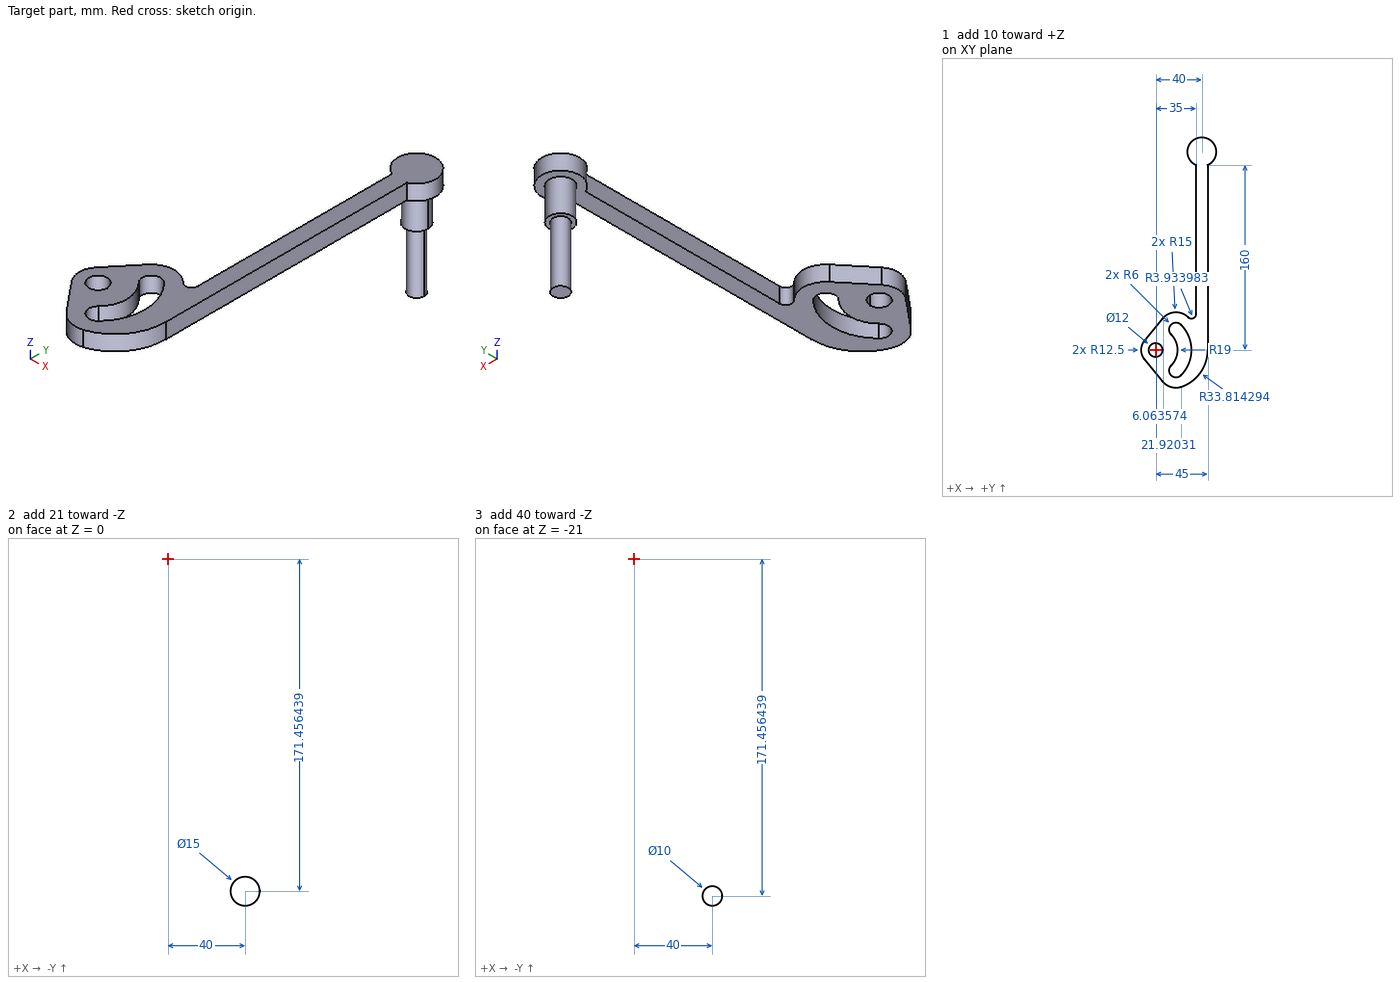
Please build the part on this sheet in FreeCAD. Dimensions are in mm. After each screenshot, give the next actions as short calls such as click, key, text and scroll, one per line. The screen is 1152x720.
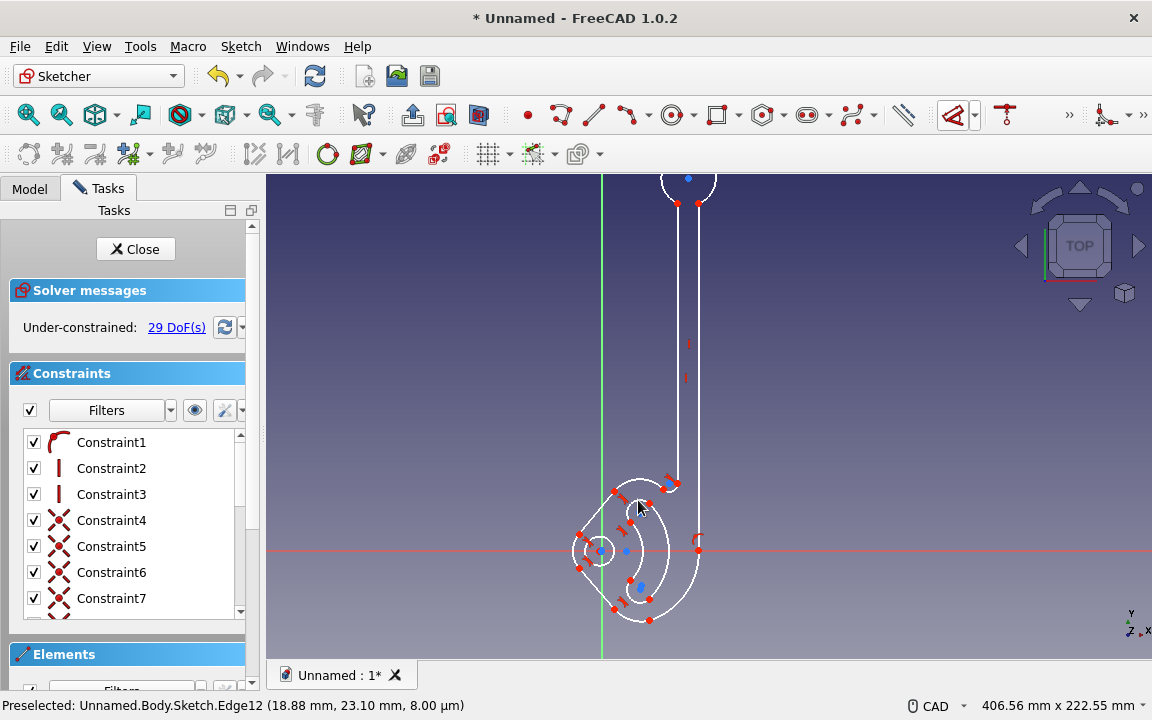
click(641, 564)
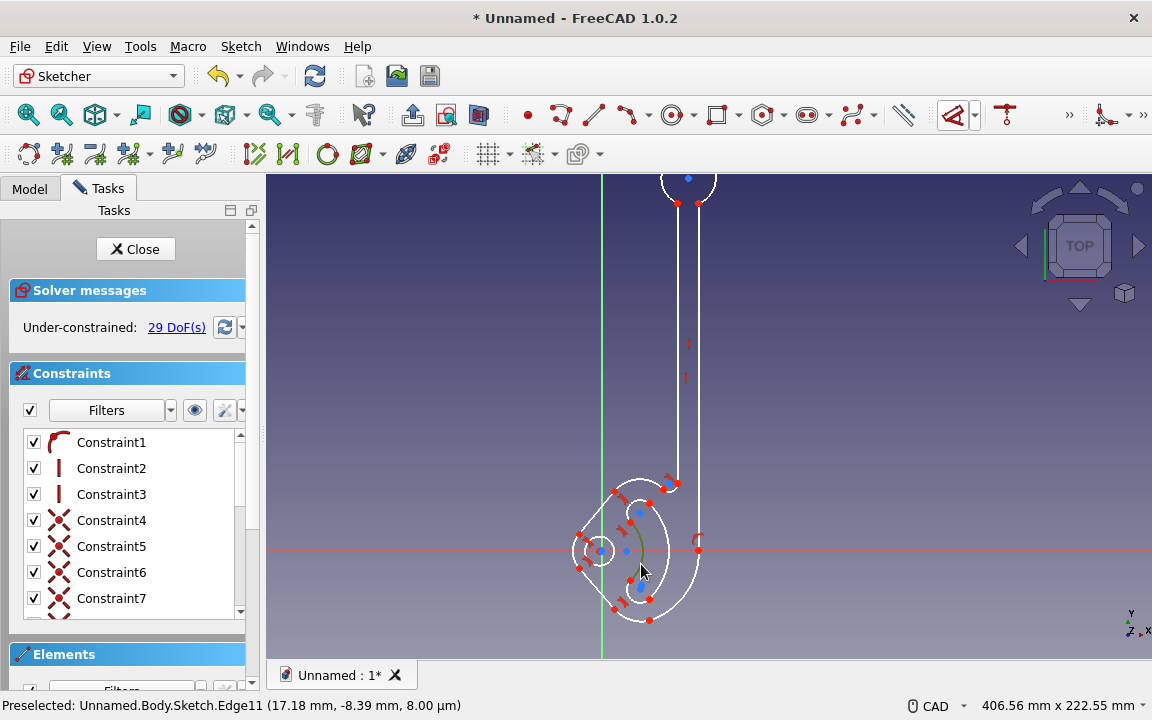
click(627, 592)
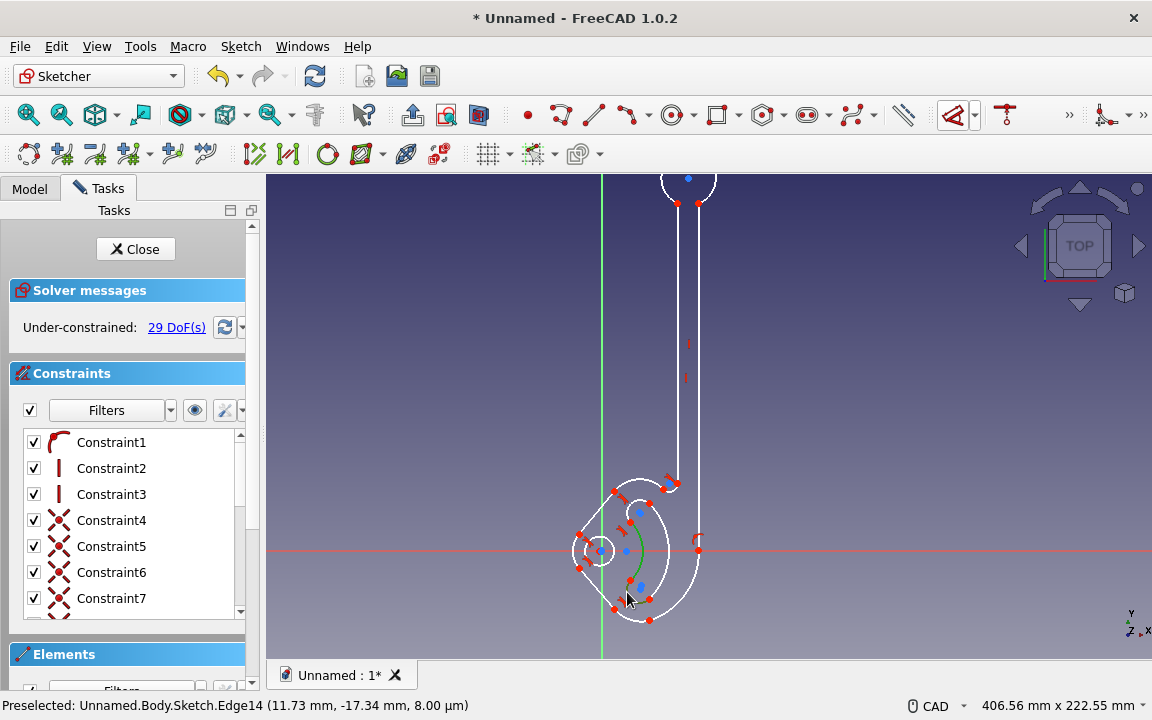
key(t)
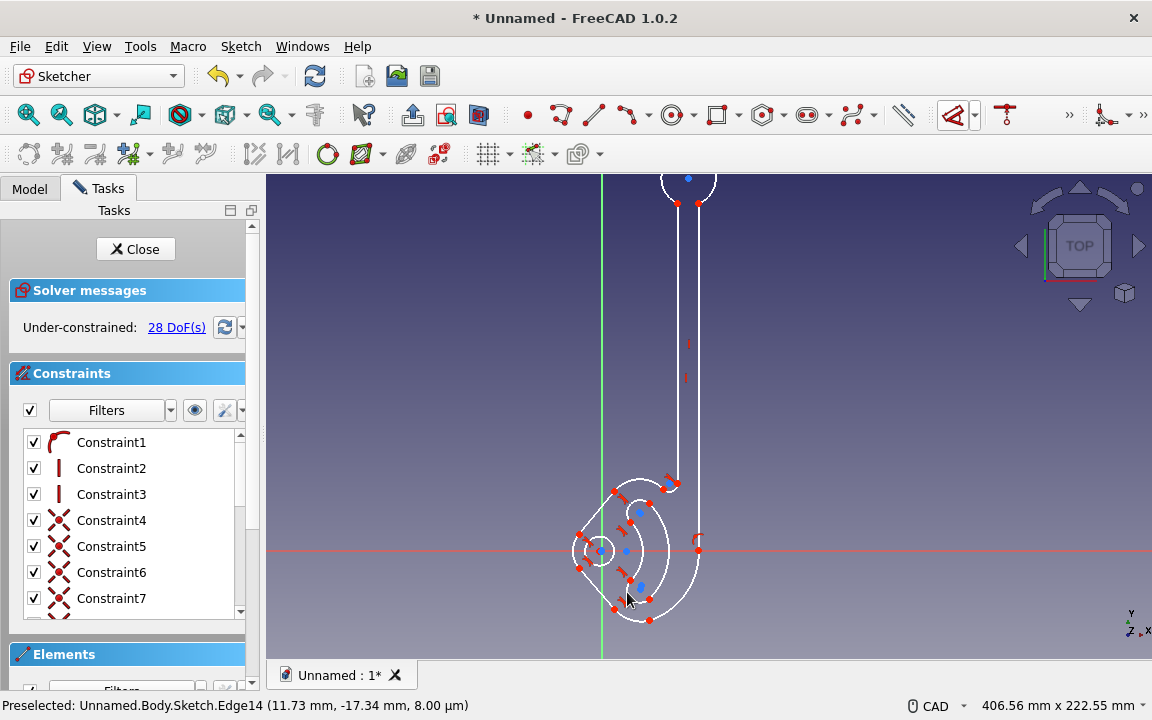
click(638, 500)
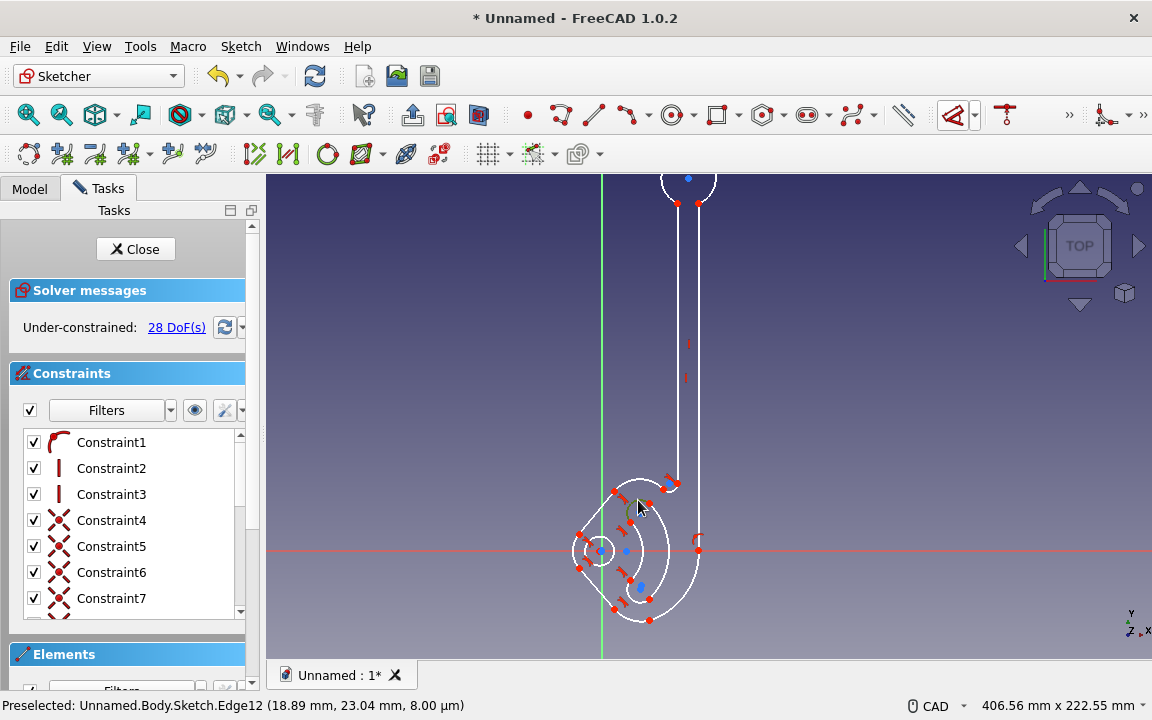
click(666, 572)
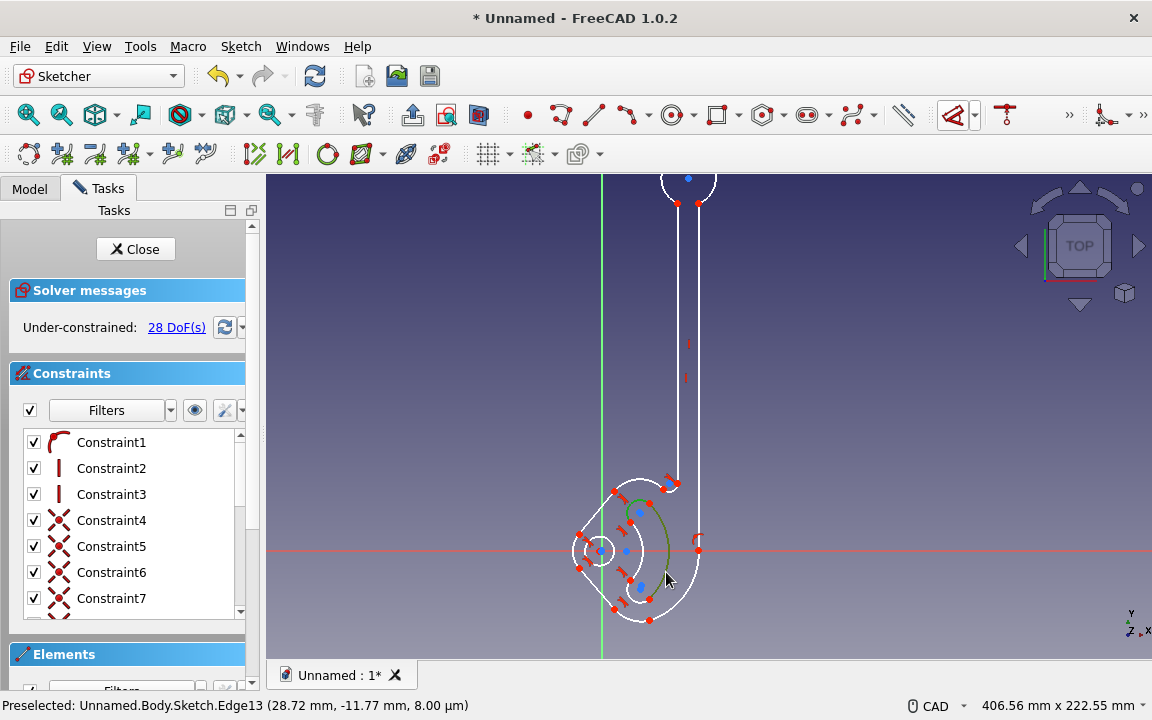
key(t)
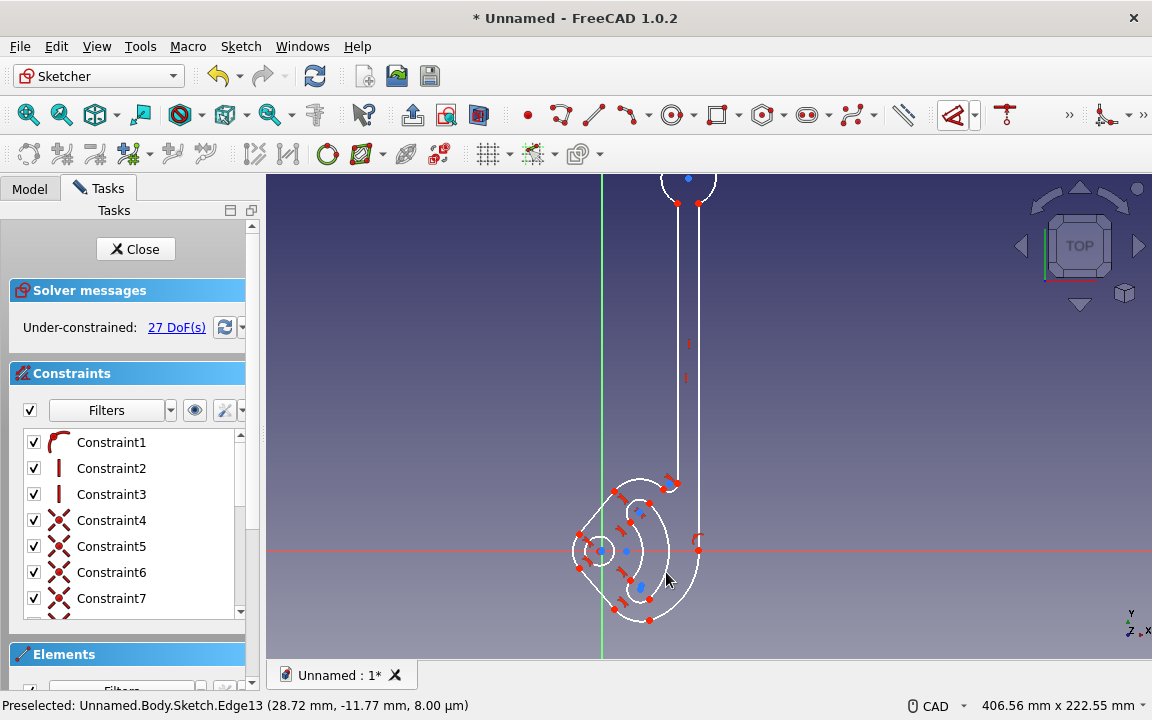
click(666, 572)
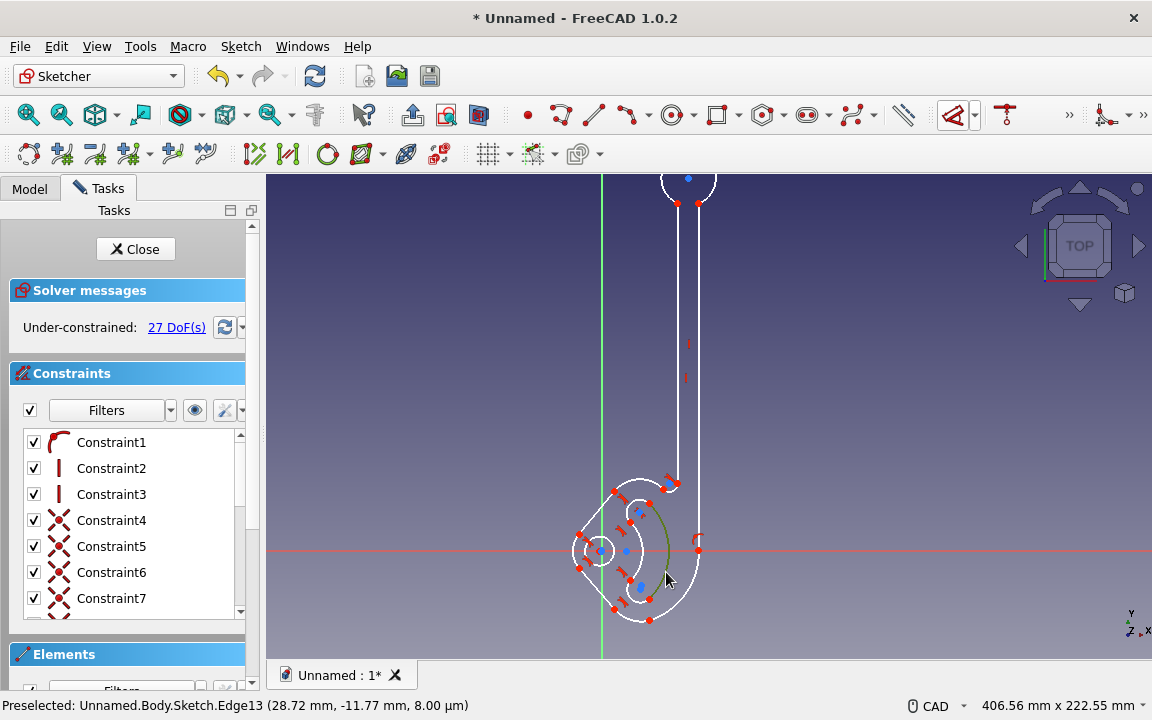
click(627, 592)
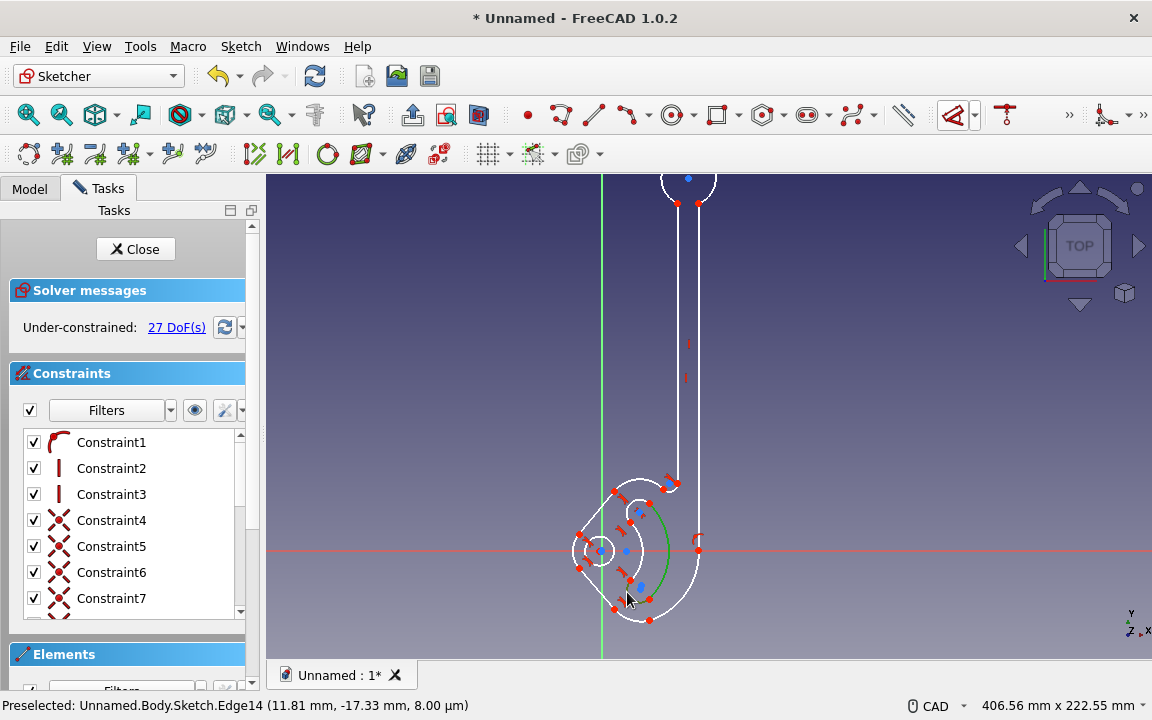
key(t)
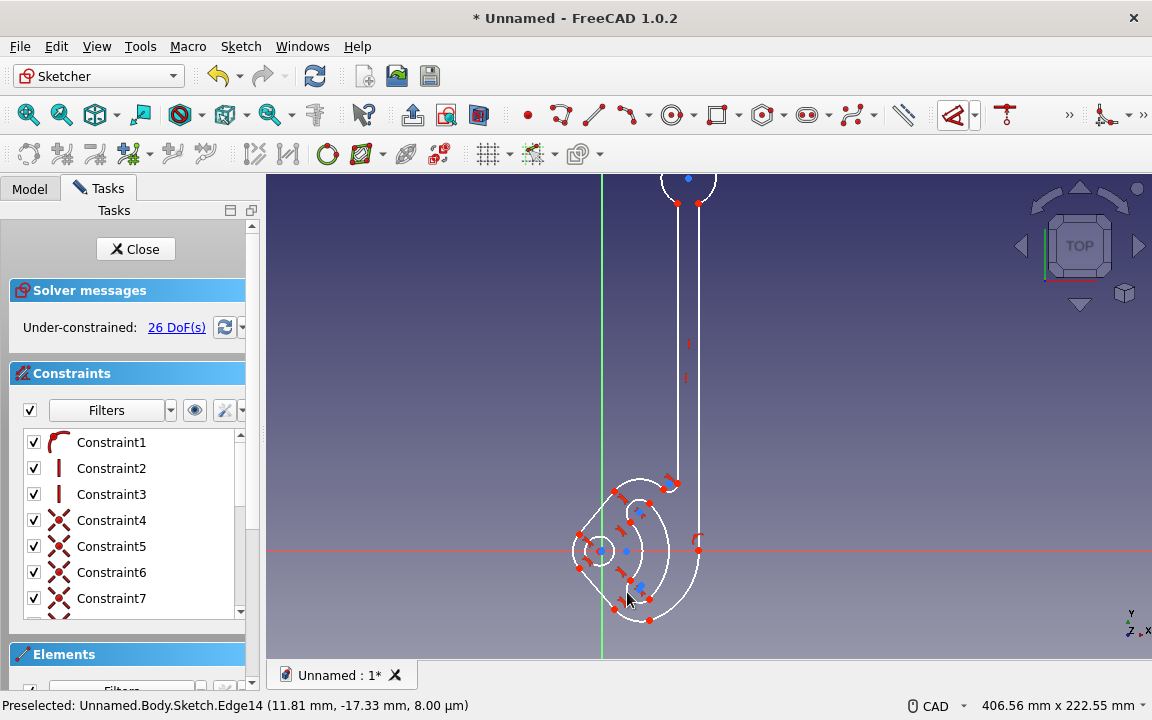
scroll(589, 541, up, 2)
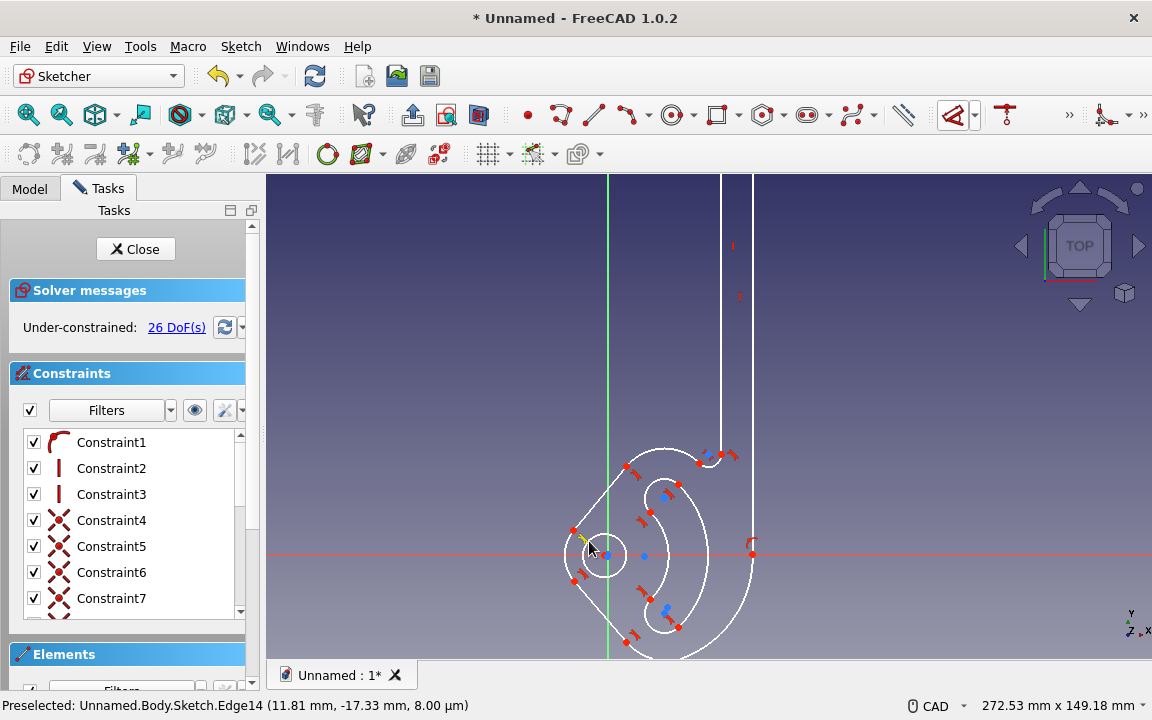
click(605, 534)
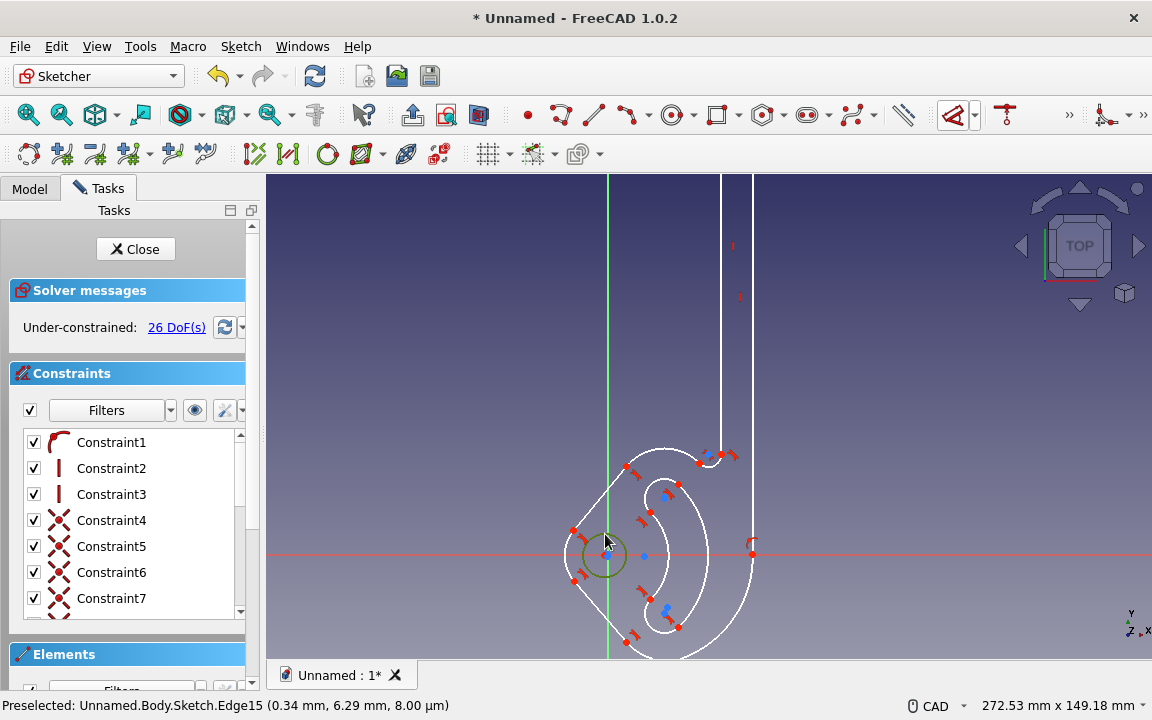
click(666, 575)